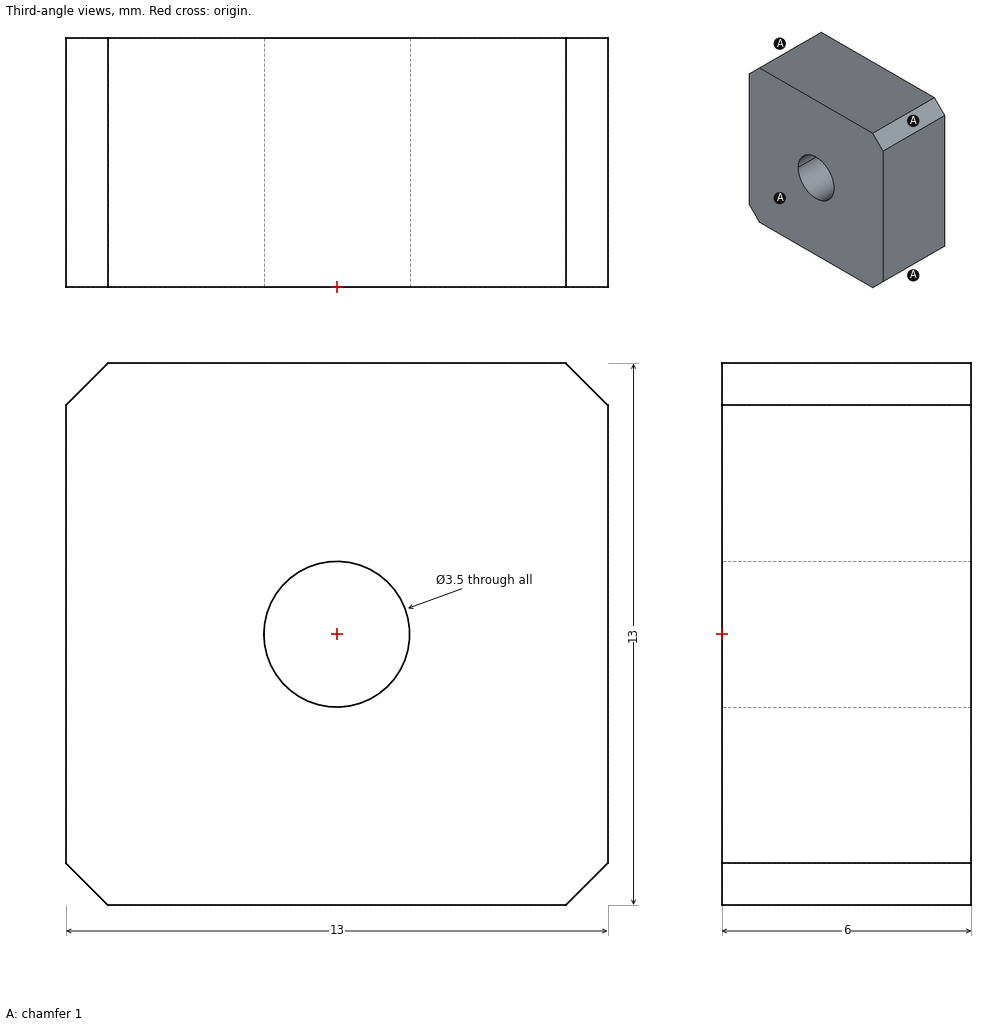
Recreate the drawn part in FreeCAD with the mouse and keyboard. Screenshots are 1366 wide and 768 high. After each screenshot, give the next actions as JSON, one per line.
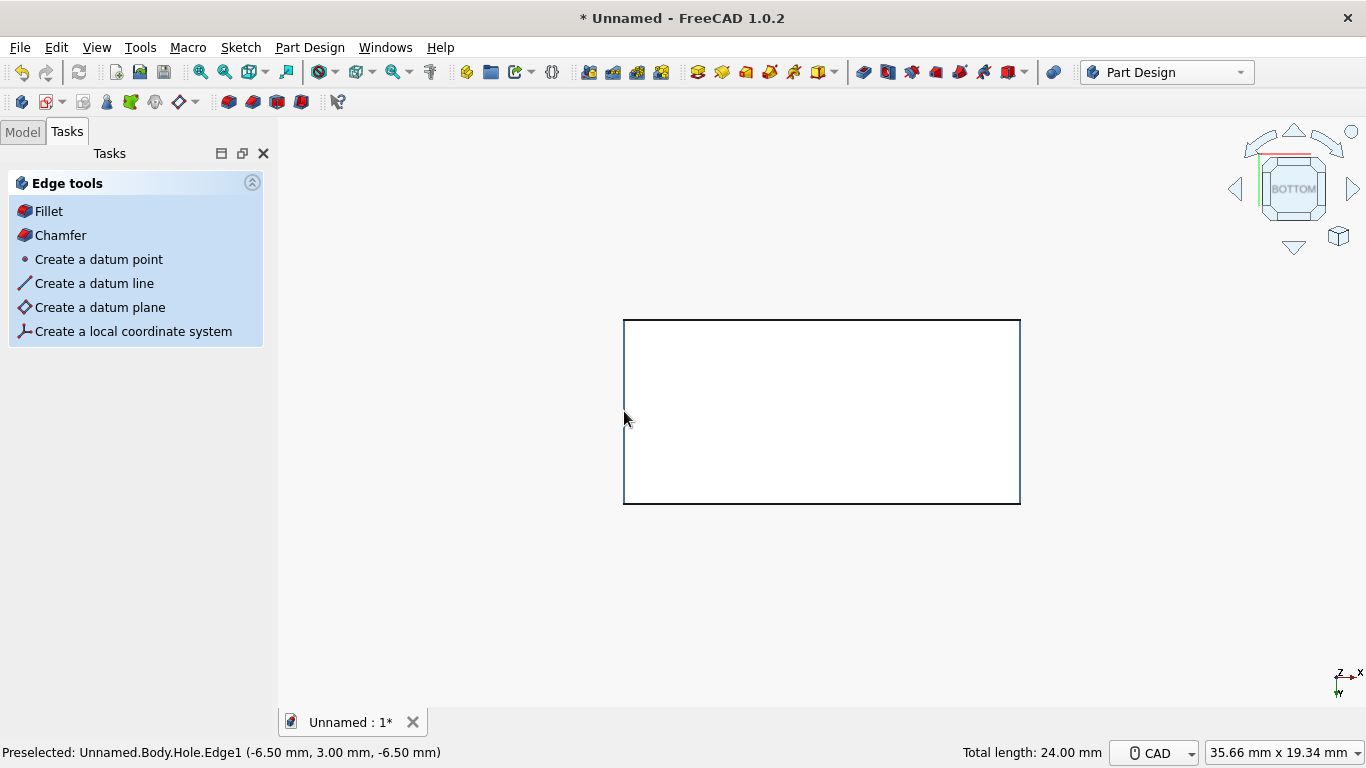
{"action": "left_click", "coordinate": [254, 102]}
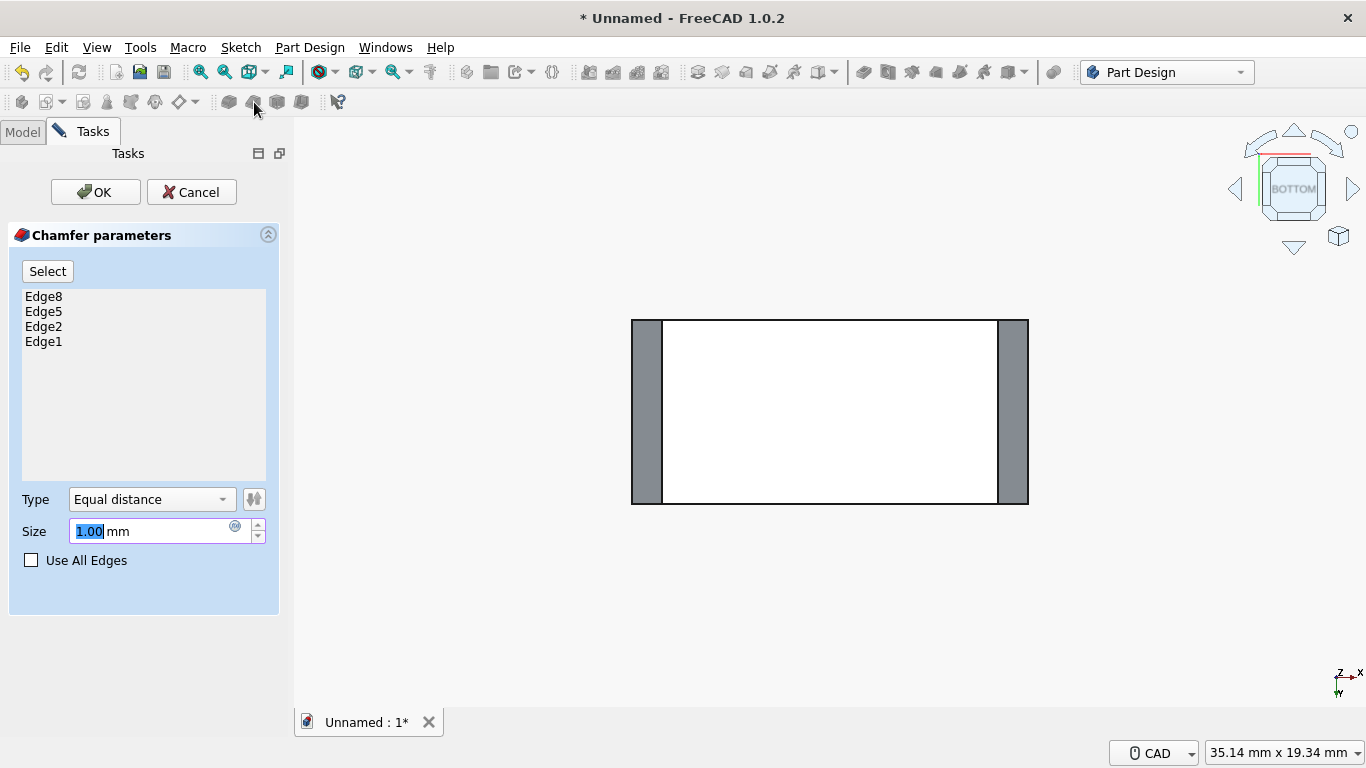
{"action": "type", "text": "1"}
{"action": "key", "text": "Tab"}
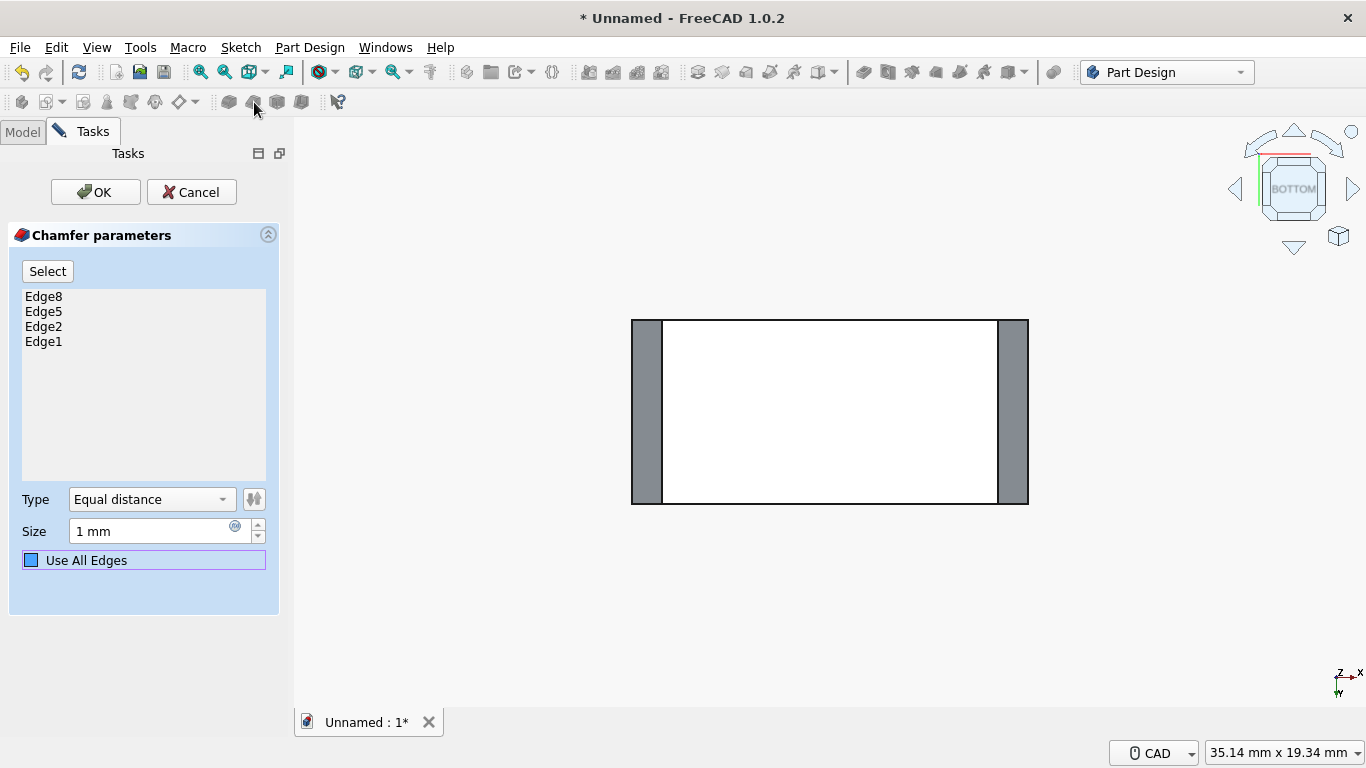
{"action": "left_click", "coordinate": [96, 192]}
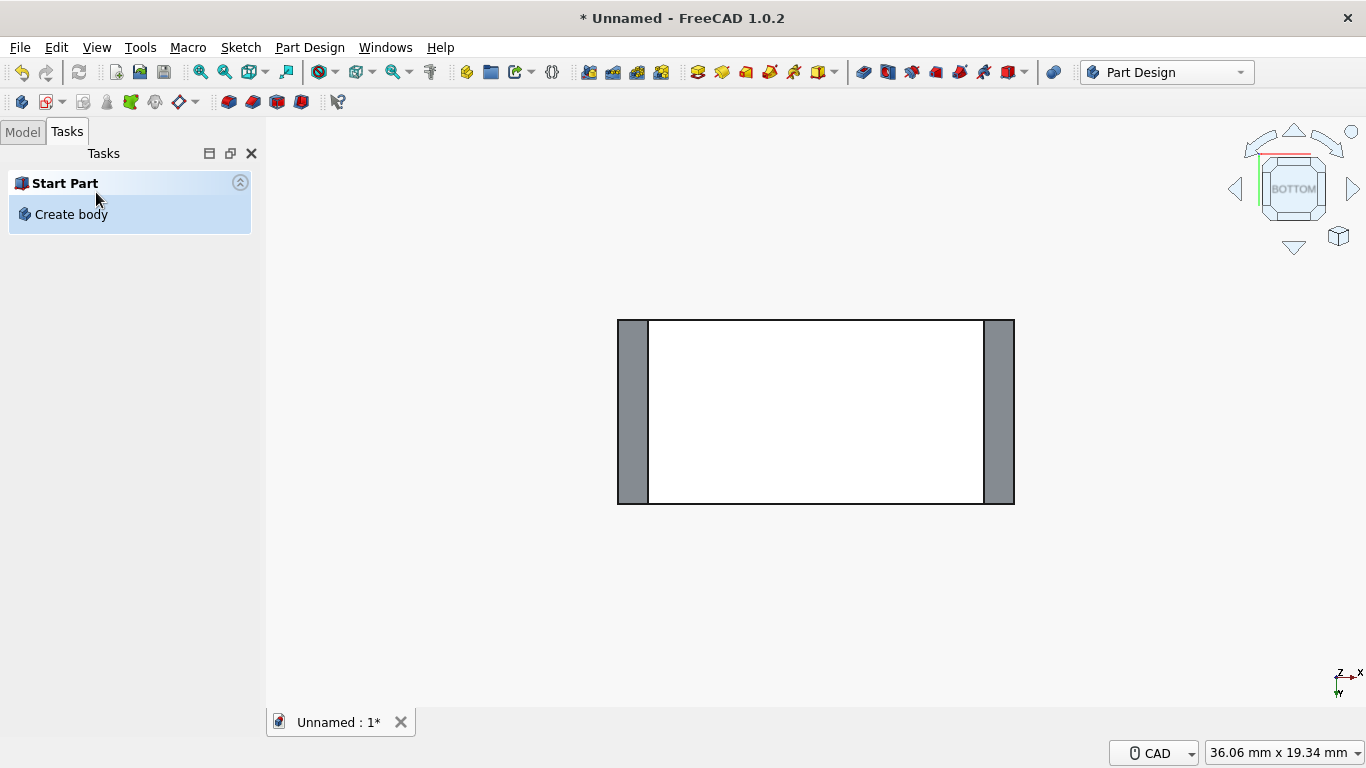
{"action": "key", "text": "0"}